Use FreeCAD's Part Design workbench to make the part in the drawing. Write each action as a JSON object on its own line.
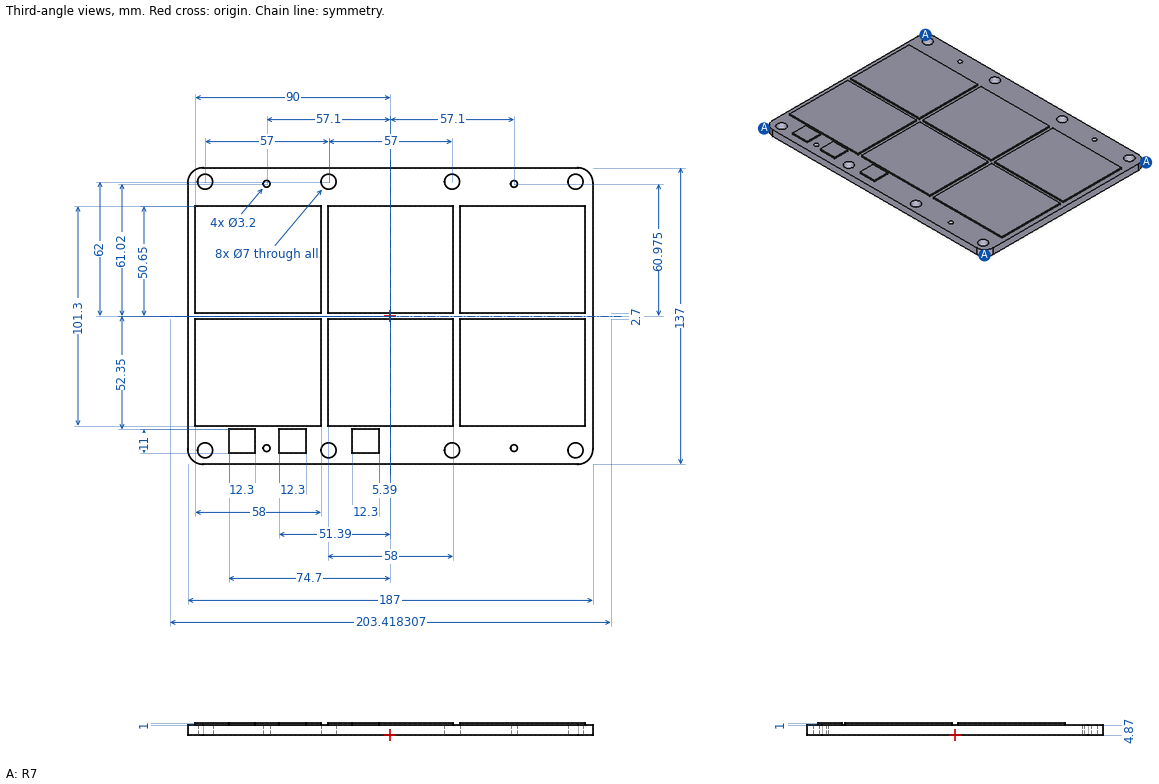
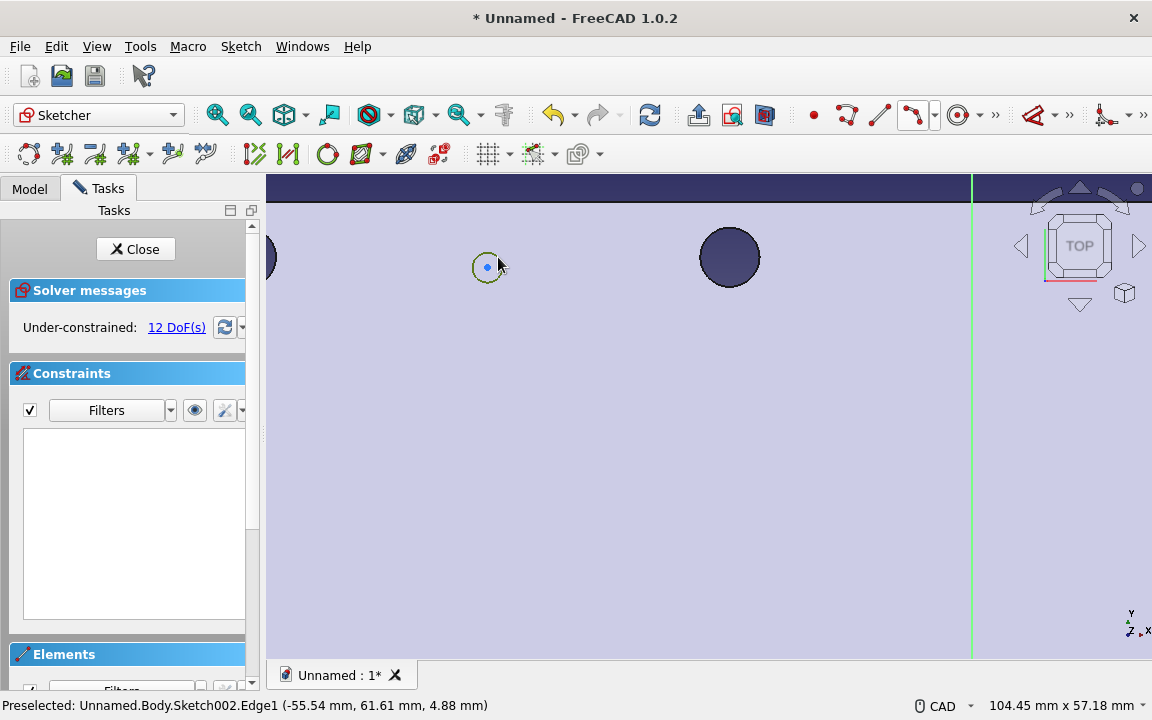
{"action": "scroll", "coordinate": [498, 258], "scroll_direction": "down", "scroll_amount": 6}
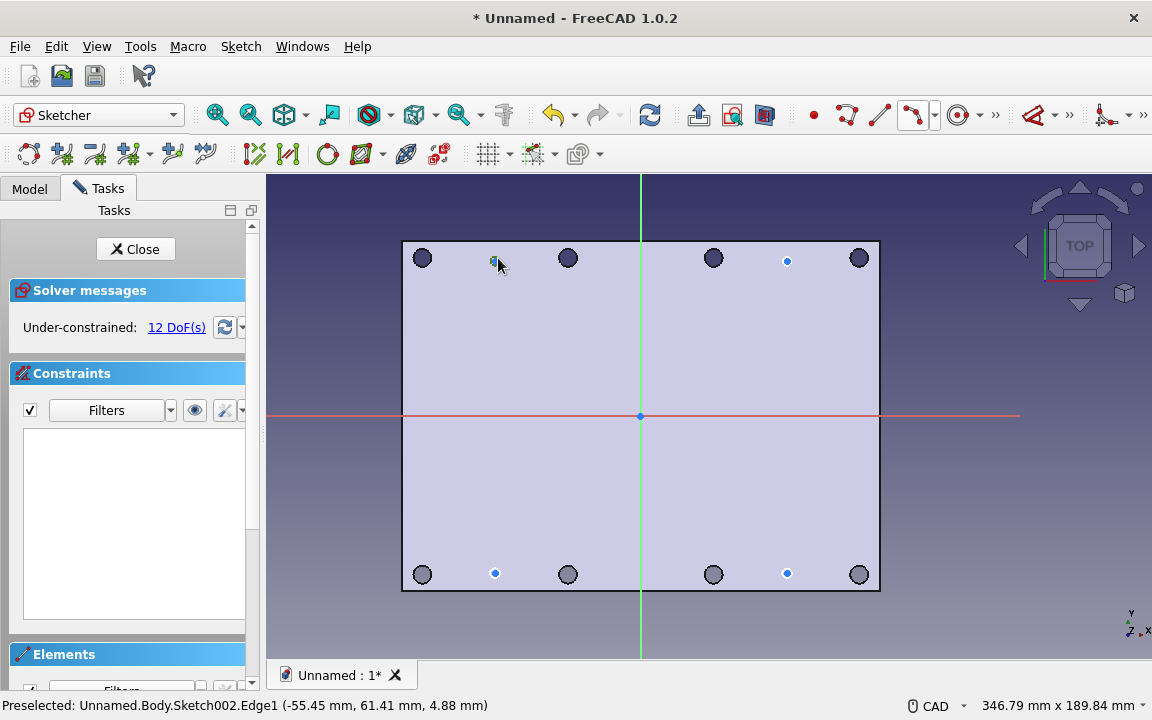
{"action": "scroll", "coordinate": [790, 258], "scroll_direction": "up", "scroll_amount": 6}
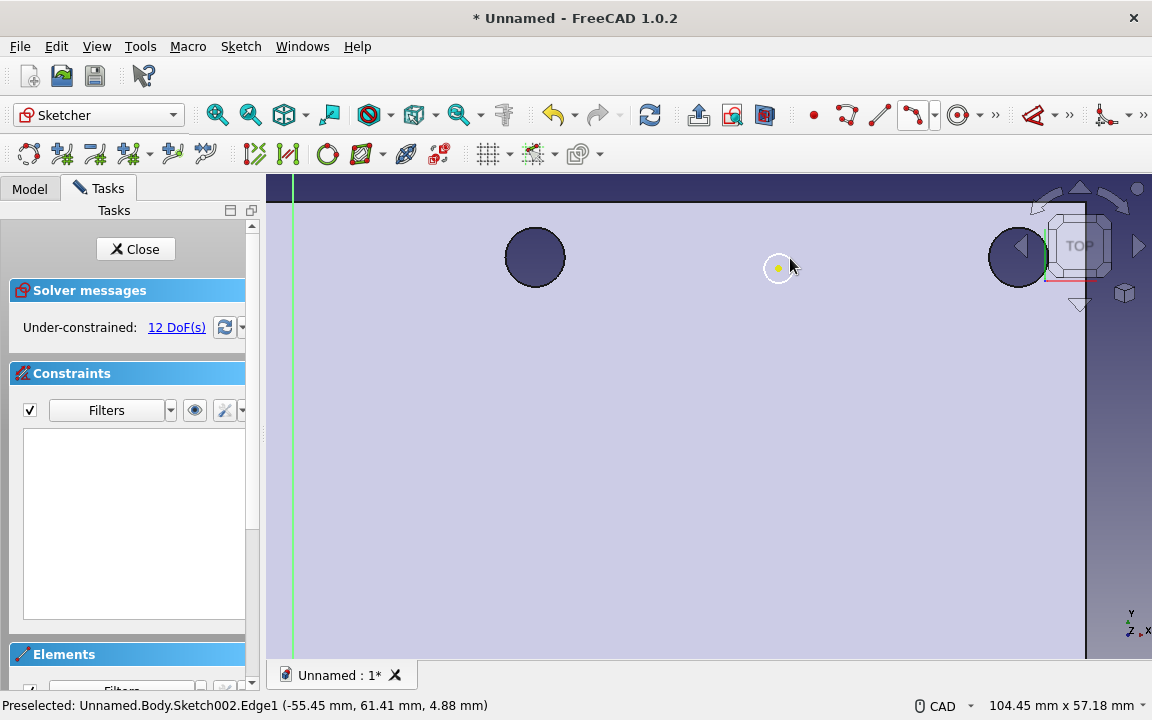
{"action": "left_click", "coordinate": [789, 258]}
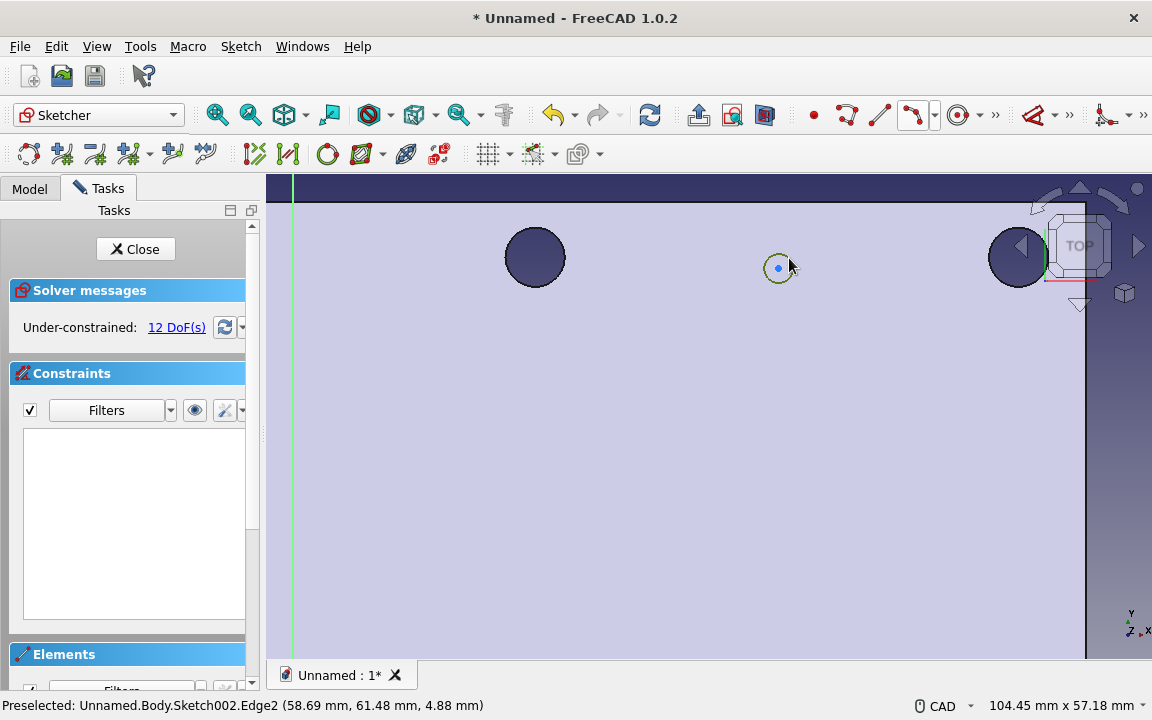
{"action": "scroll", "coordinate": [790, 258], "scroll_direction": "down", "scroll_amount": 6}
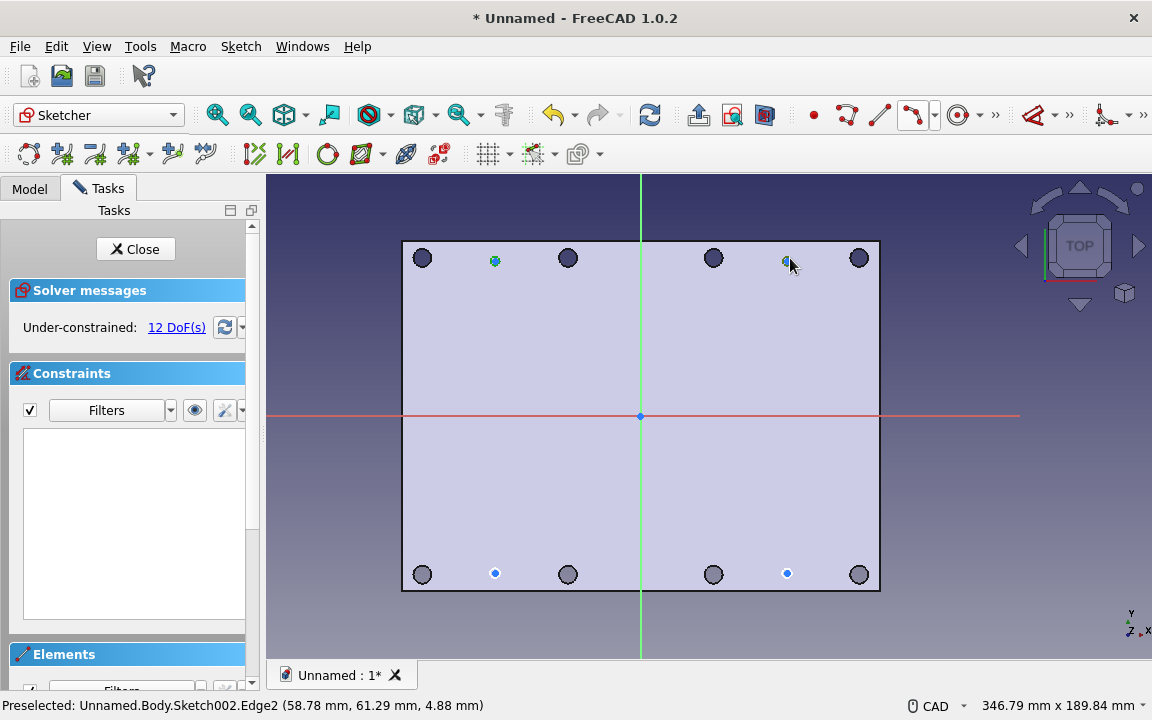
{"action": "scroll", "coordinate": [790, 570], "scroll_direction": "up", "scroll_amount": 6}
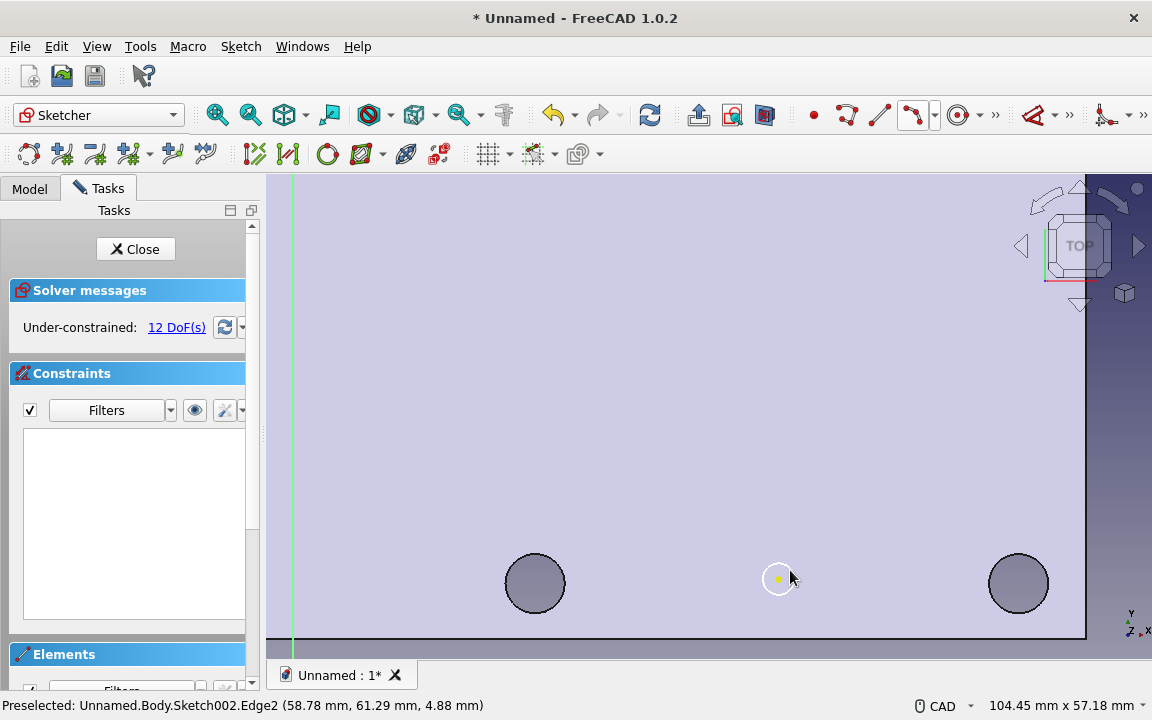
{"action": "left_click", "coordinate": [790, 568]}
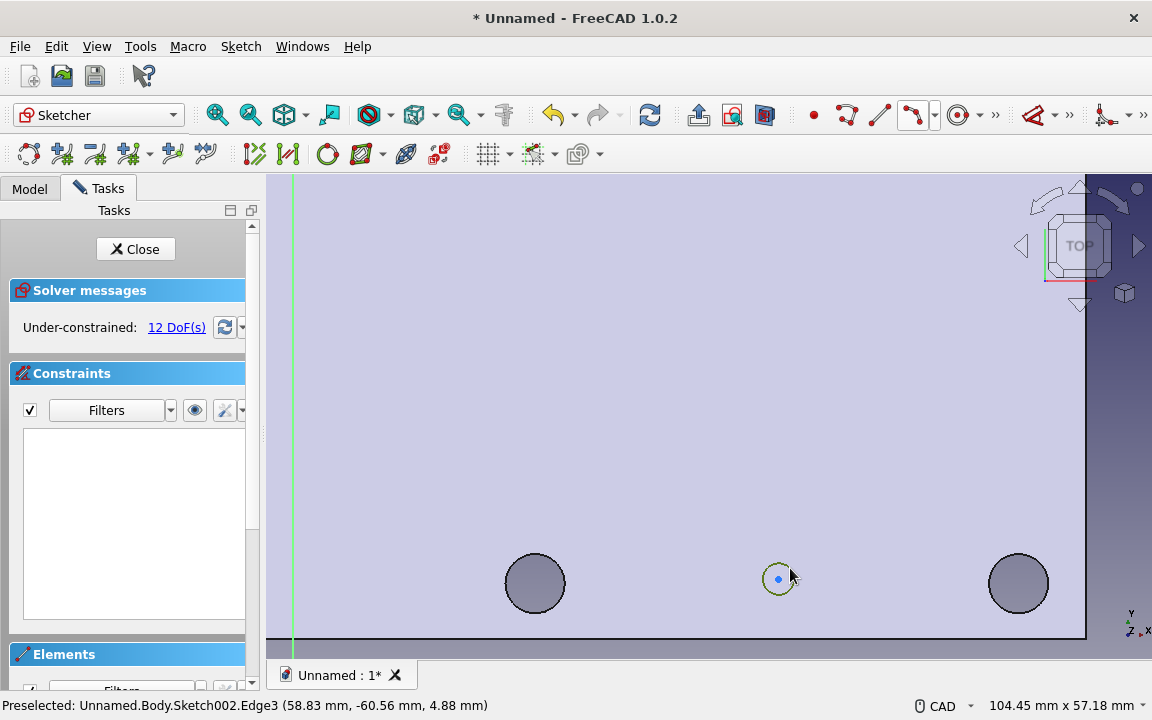
{"action": "scroll", "coordinate": [790, 571], "scroll_direction": "down", "scroll_amount": 6}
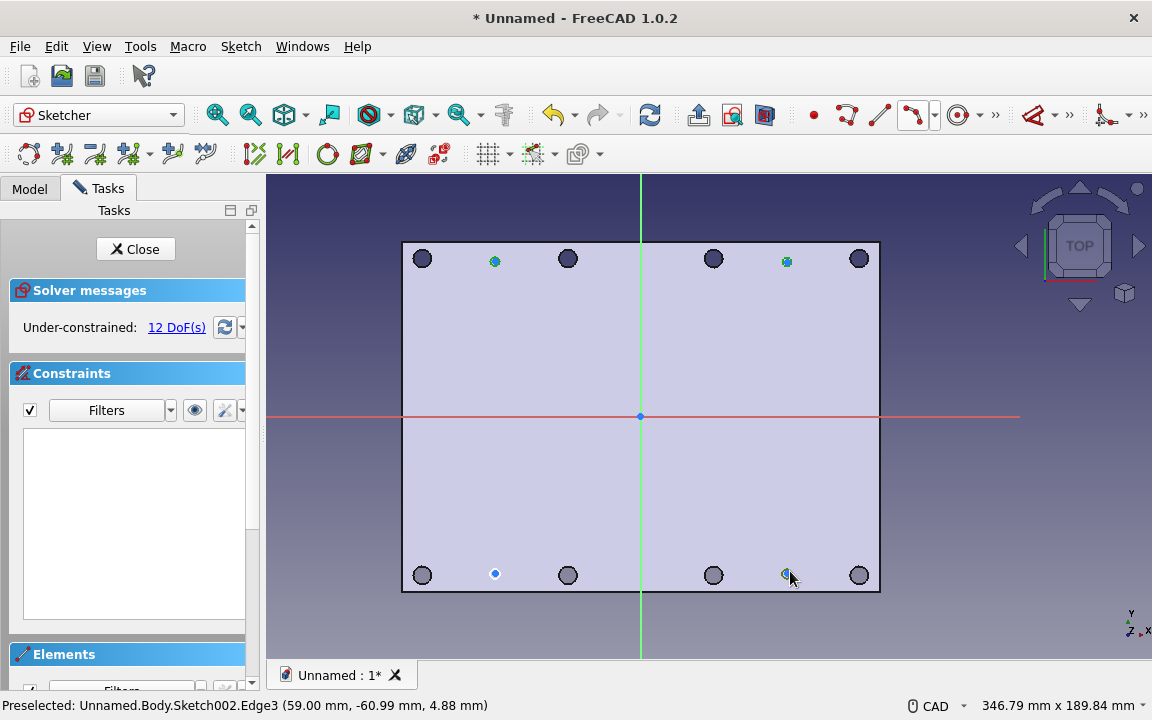
{"action": "scroll", "coordinate": [498, 571], "scroll_direction": "up", "scroll_amount": 6}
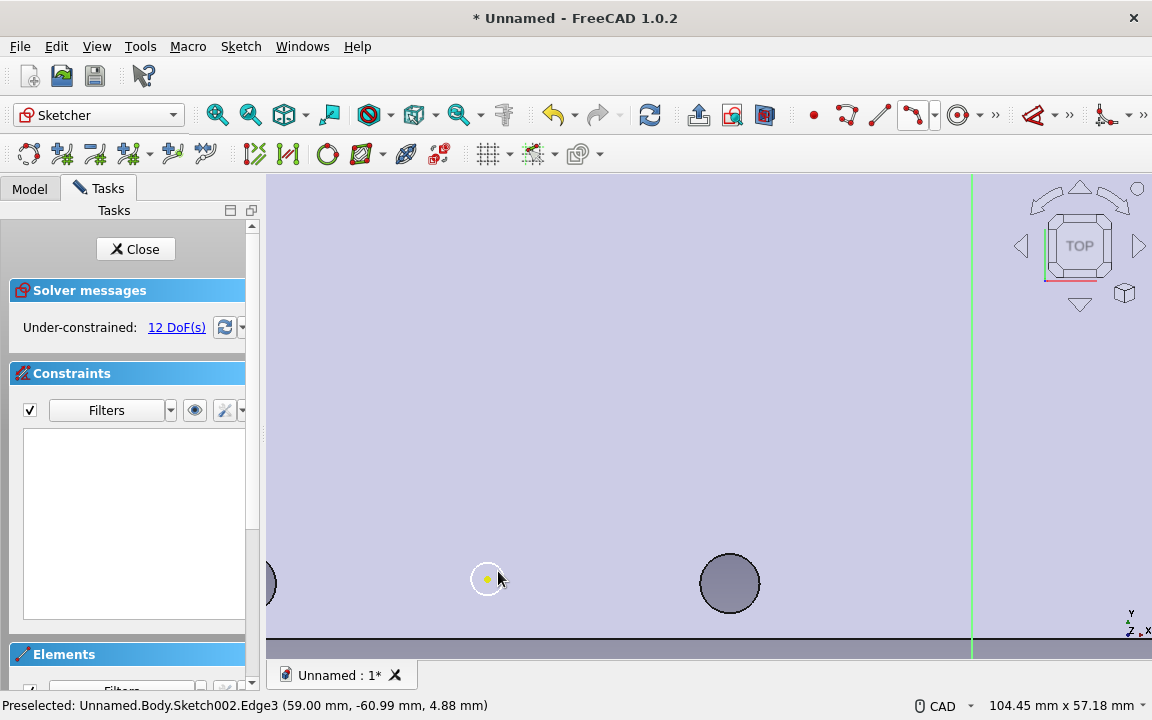
{"action": "left_click", "coordinate": [499, 568]}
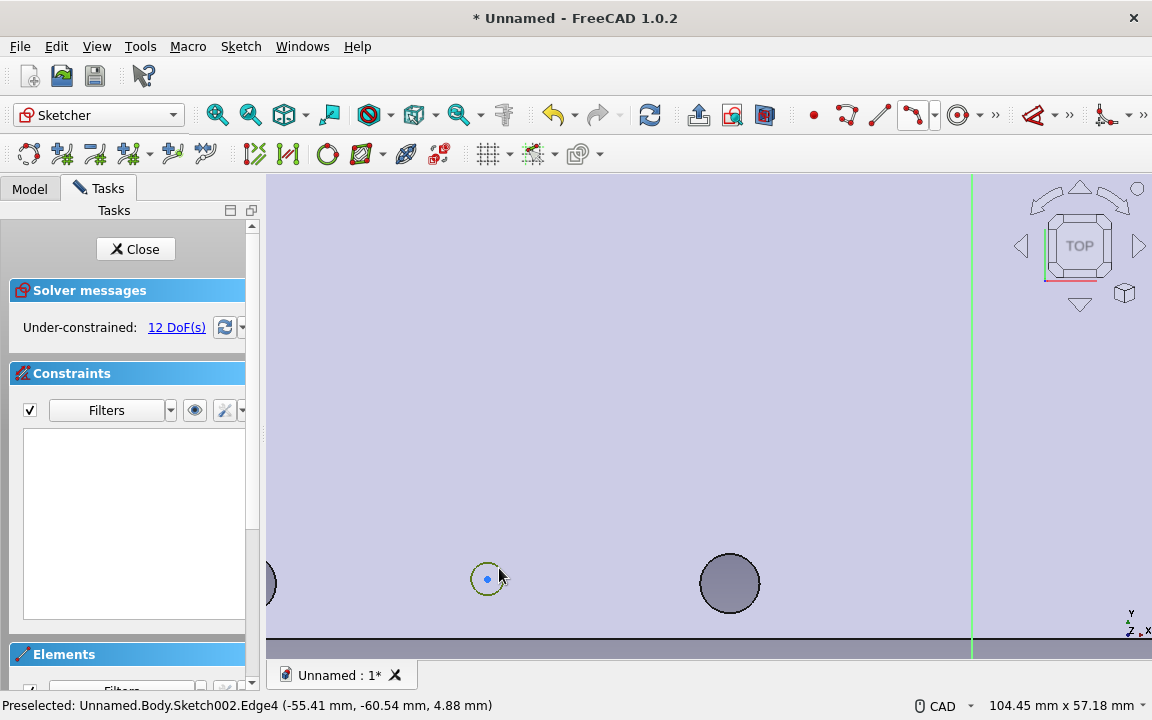
{"action": "key", "text": "e"}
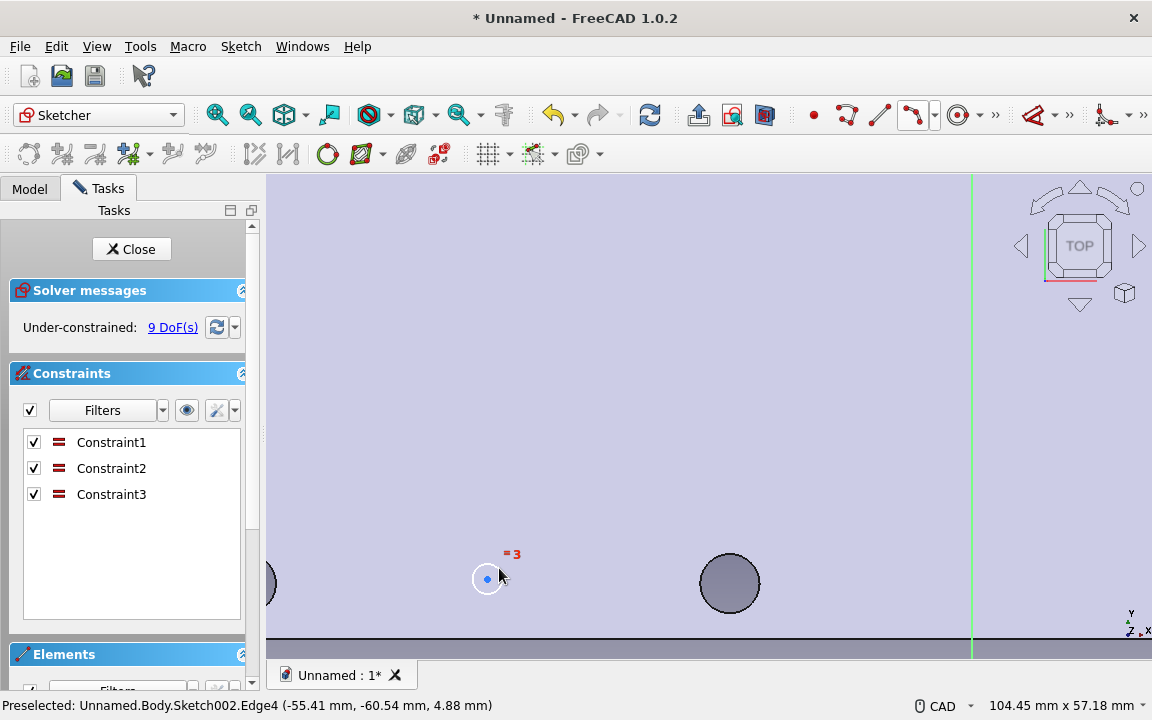
{"action": "scroll", "coordinate": [498, 571], "scroll_direction": "down", "scroll_amount": 6}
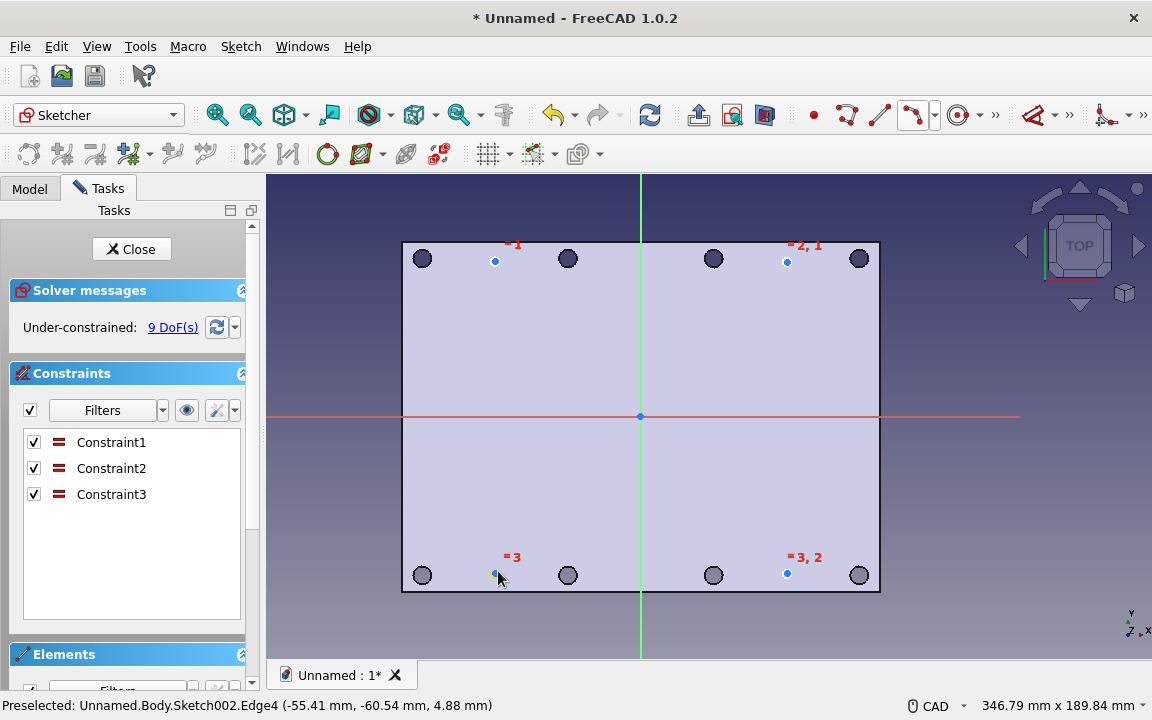
{"action": "left_click", "coordinate": [787, 262]}